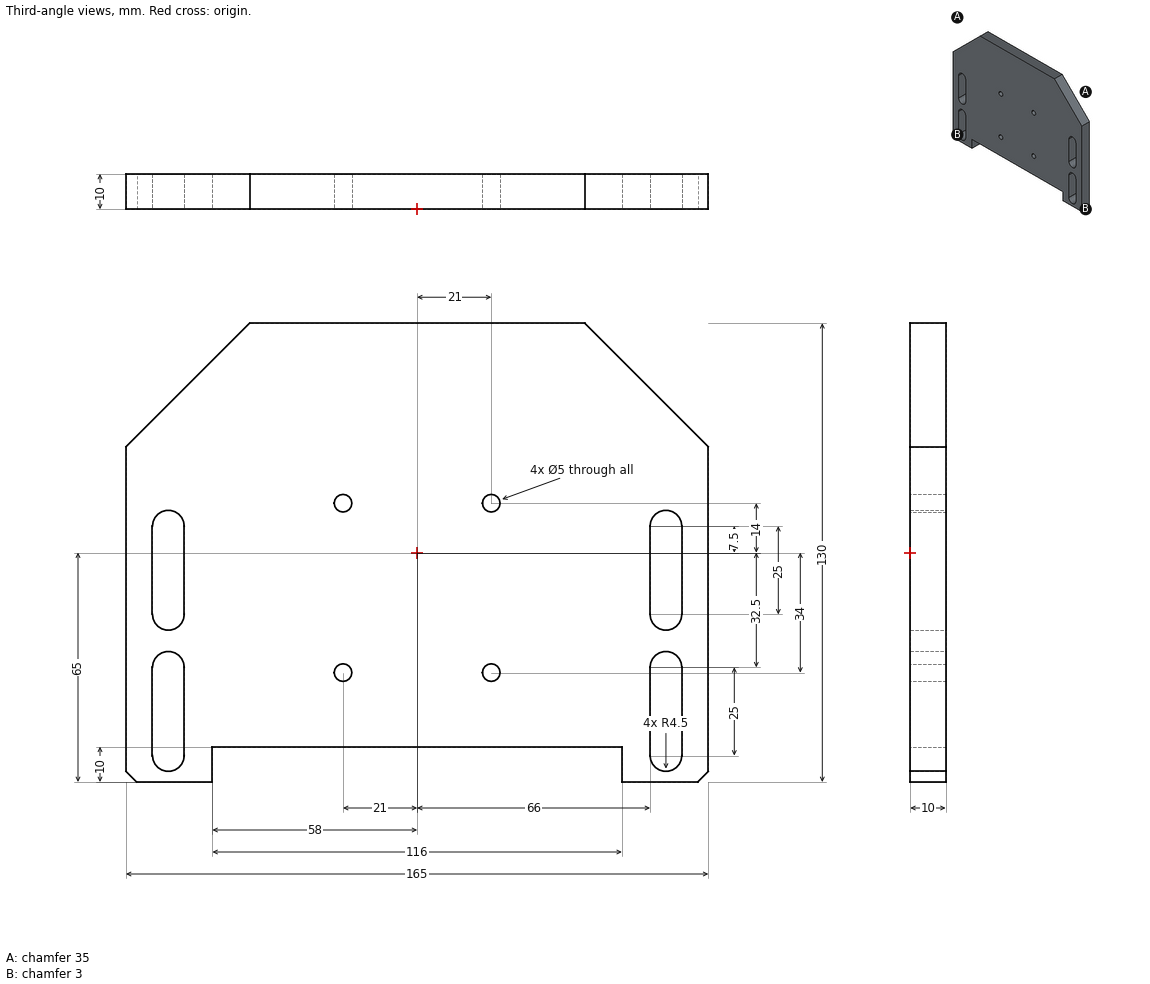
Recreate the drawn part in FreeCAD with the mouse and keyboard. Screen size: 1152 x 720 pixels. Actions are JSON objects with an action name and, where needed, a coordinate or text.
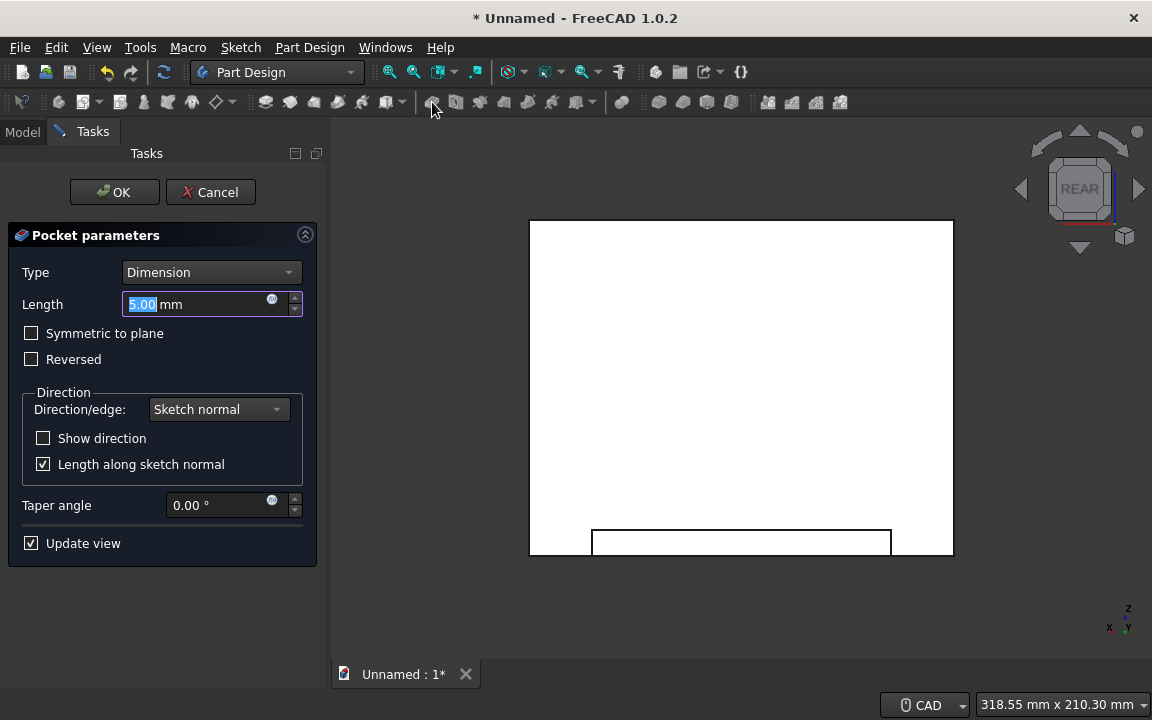
{"action": "type", "text": "10"}
{"action": "key", "text": "Tab"}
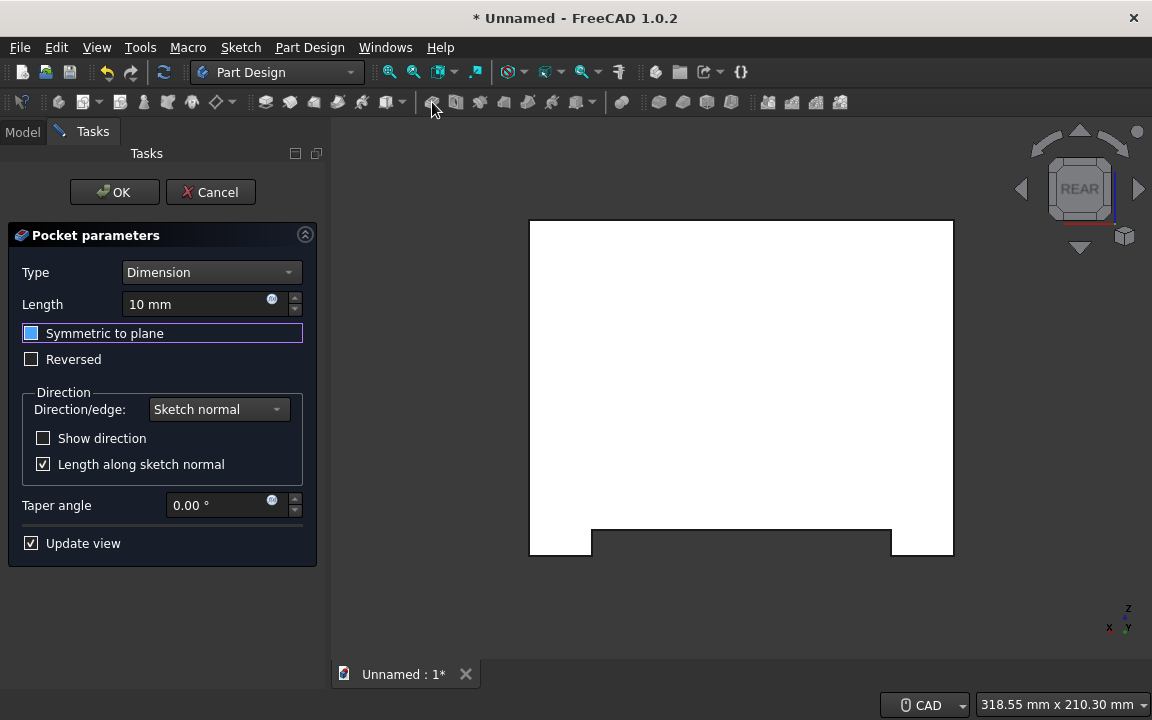
{"action": "left_click", "coordinate": [115, 192]}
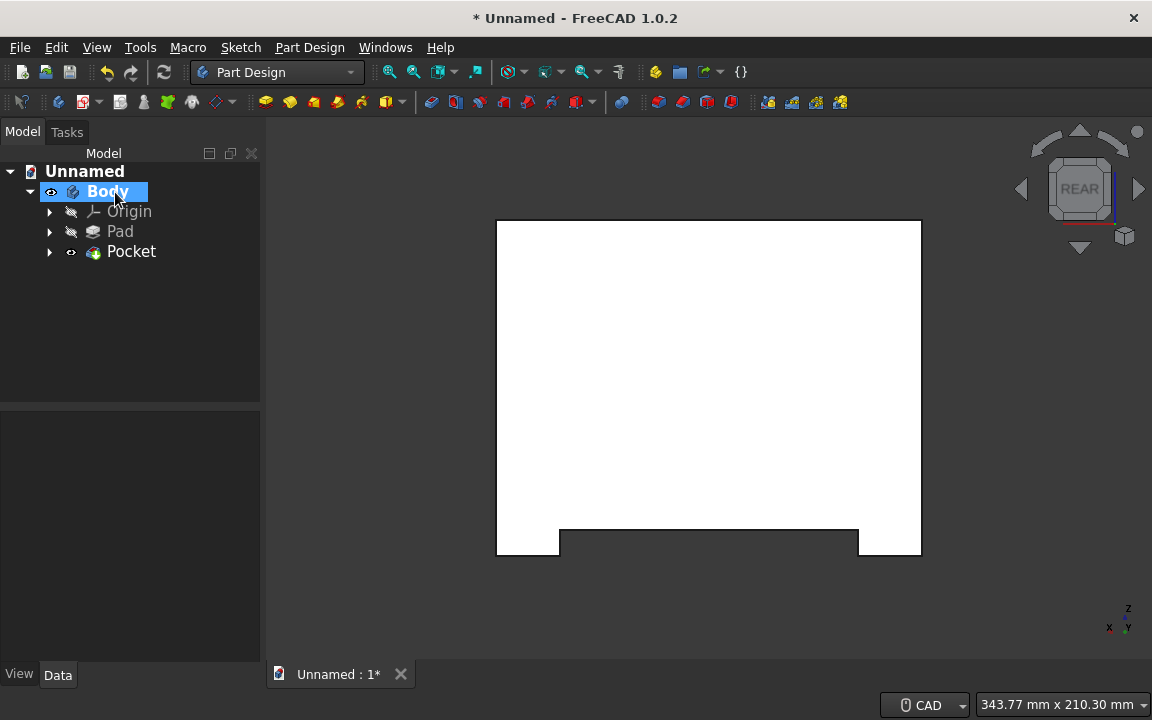
{"action": "left_click", "coordinate": [648, 387]}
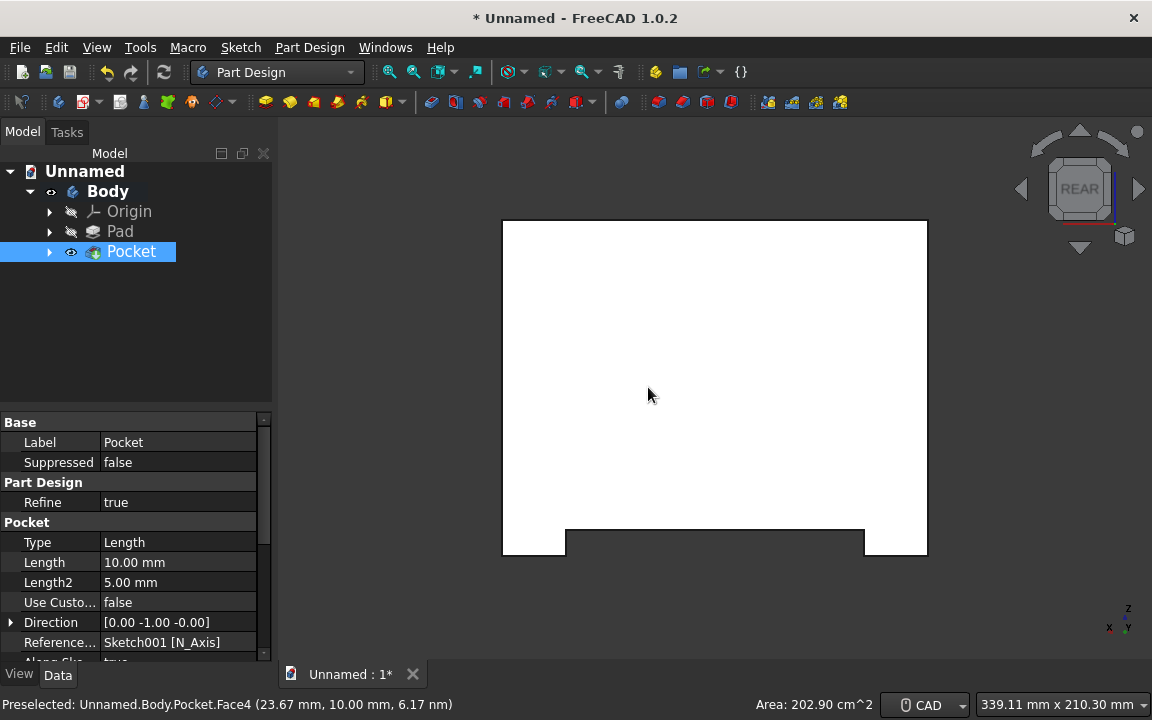
{"action": "left_click", "coordinate": [84, 102]}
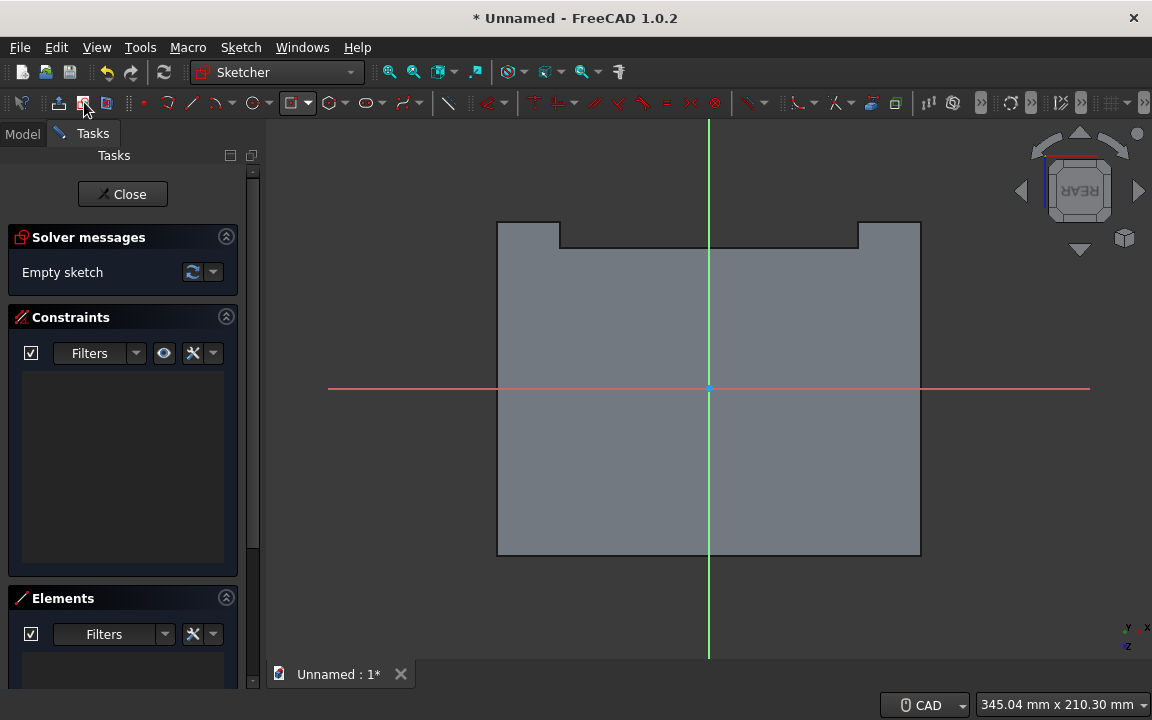
{"action": "scroll", "coordinate": [987, 247], "scroll_direction": "up", "scroll_amount": 3}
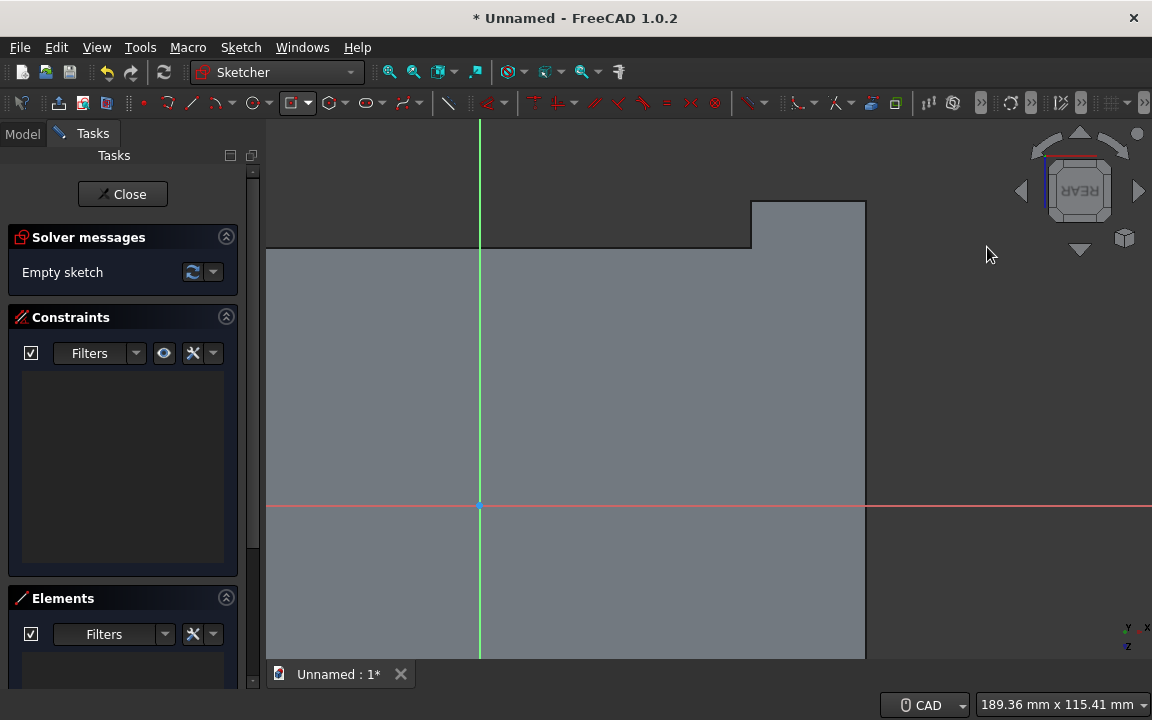
{"action": "key", "text": "g s"}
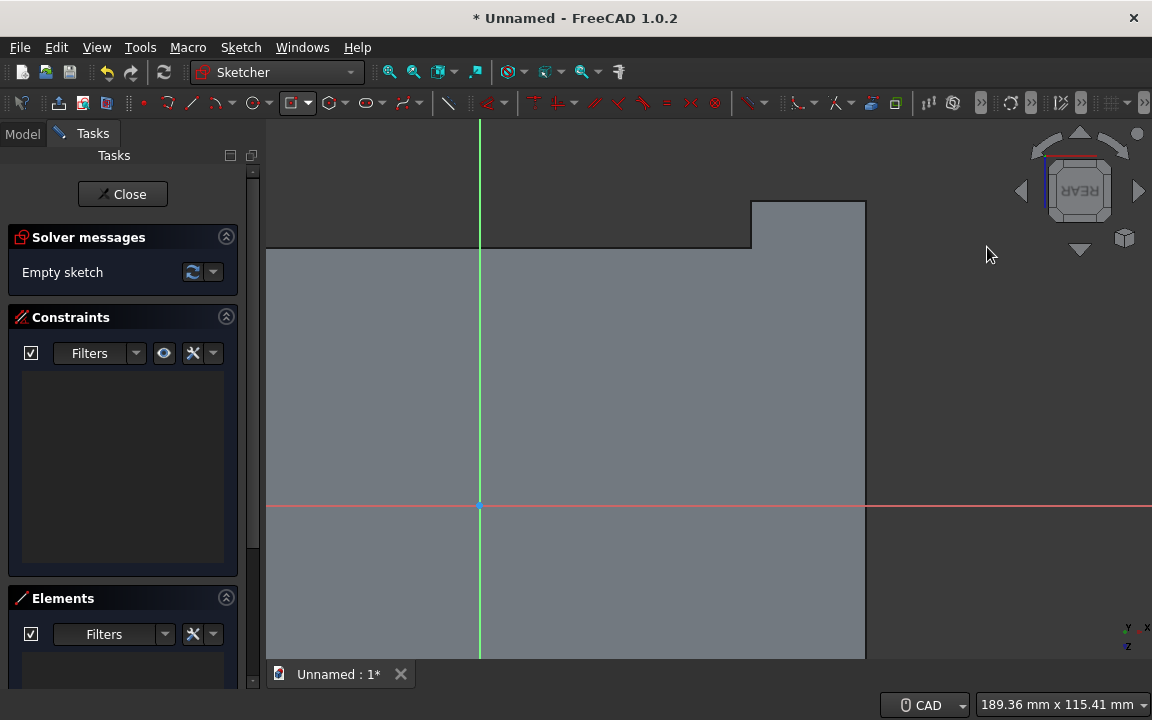
{"action": "left_click", "coordinate": [810, 353]}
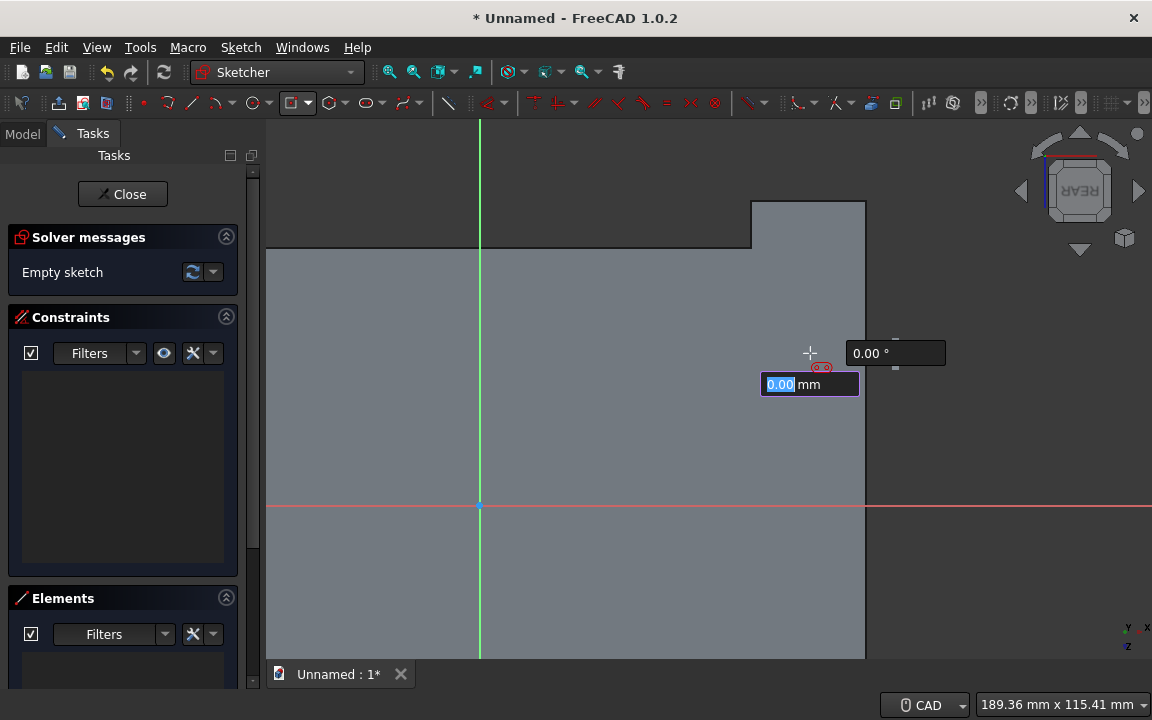
{"action": "left_click", "coordinate": [810, 237]}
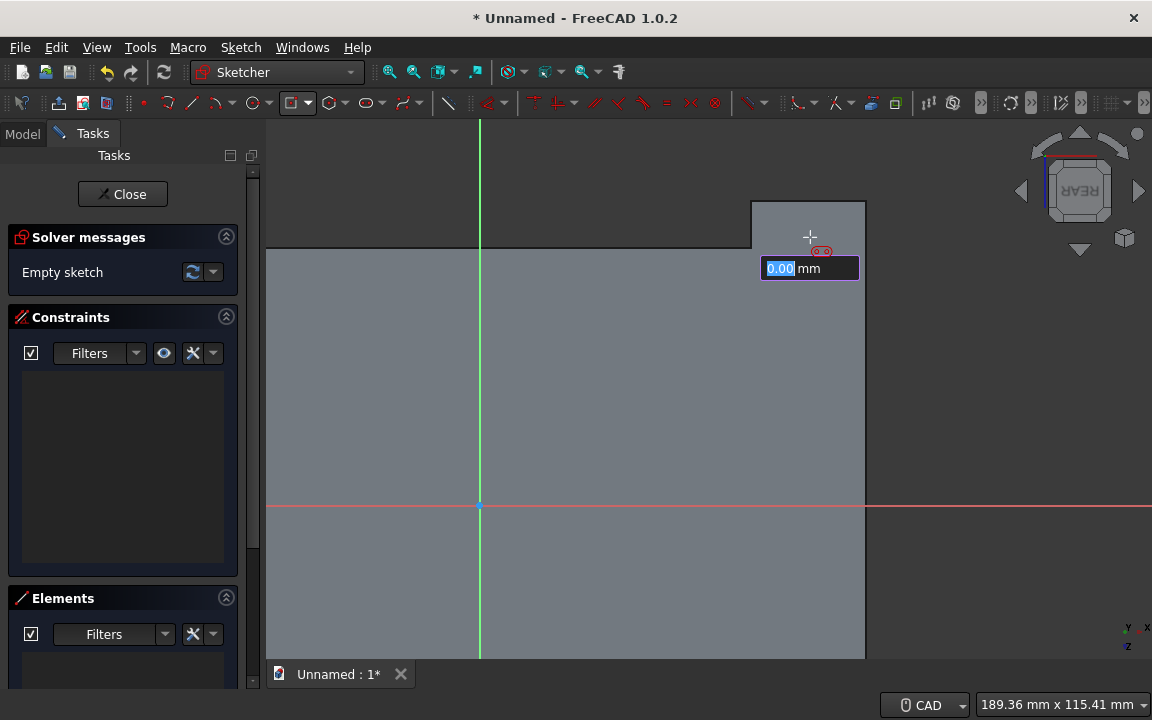
{"action": "left_click", "coordinate": [831, 295]}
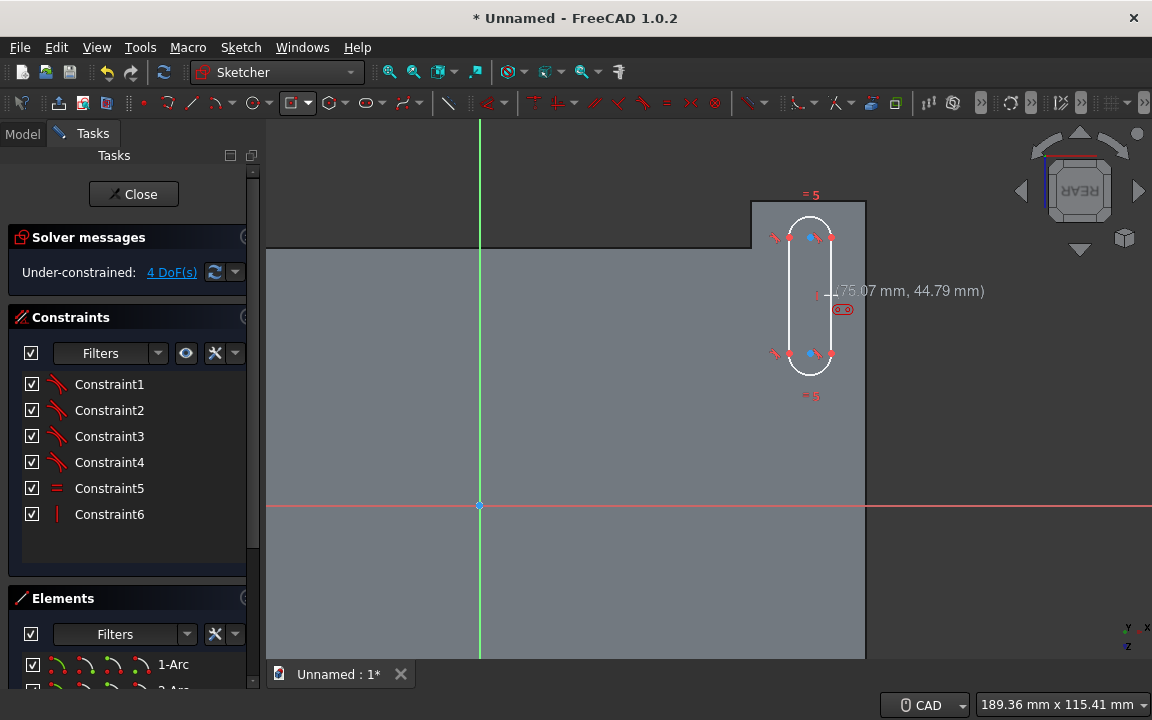
{"action": "left_click", "coordinate": [810, 541]}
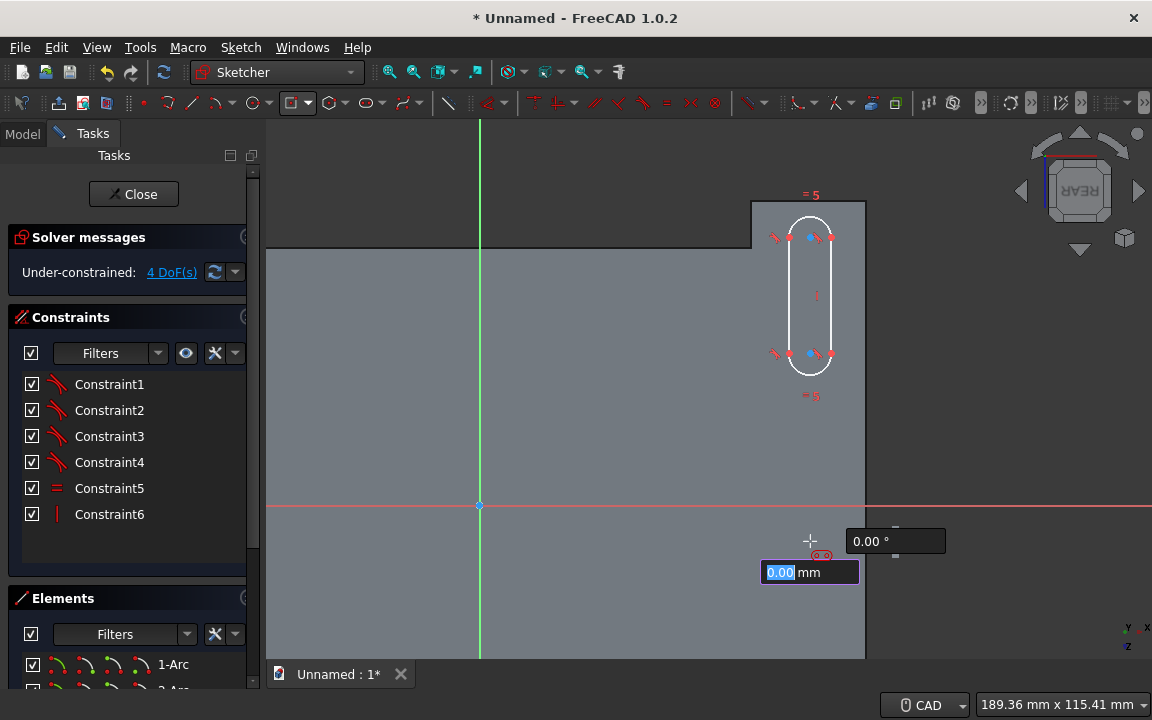
{"action": "left_click", "coordinate": [810, 424]}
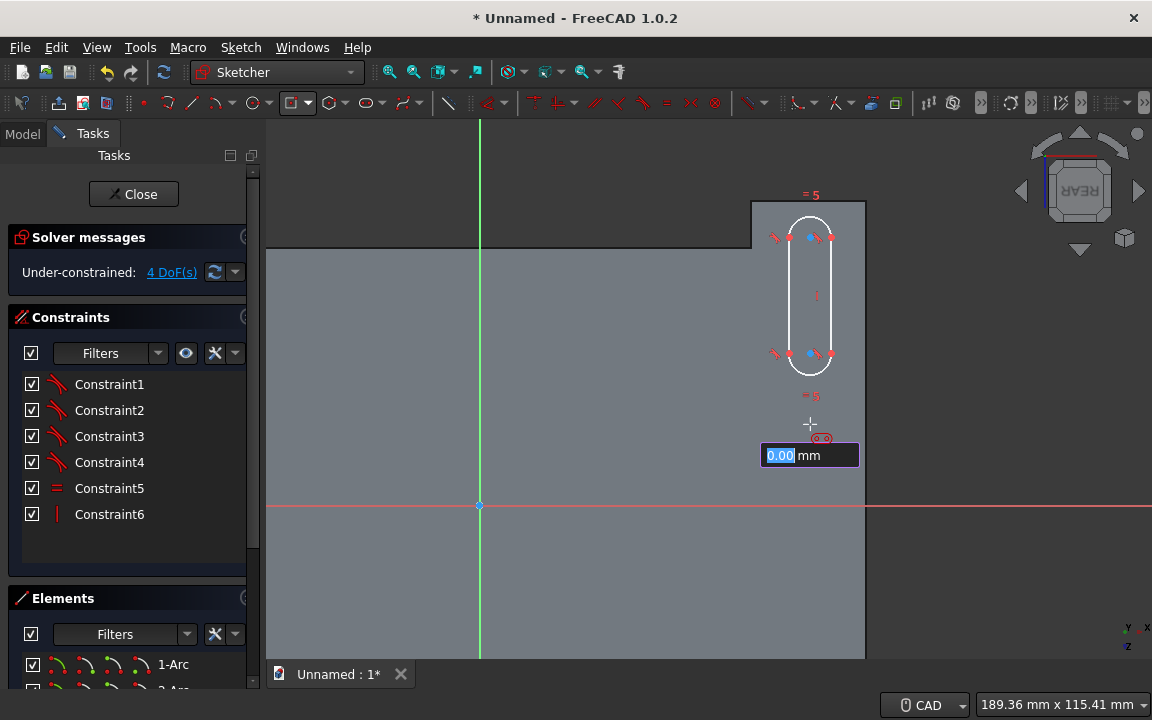
{"action": "left_click", "coordinate": [831, 482]}
{"action": "key", "text": "Escape"}